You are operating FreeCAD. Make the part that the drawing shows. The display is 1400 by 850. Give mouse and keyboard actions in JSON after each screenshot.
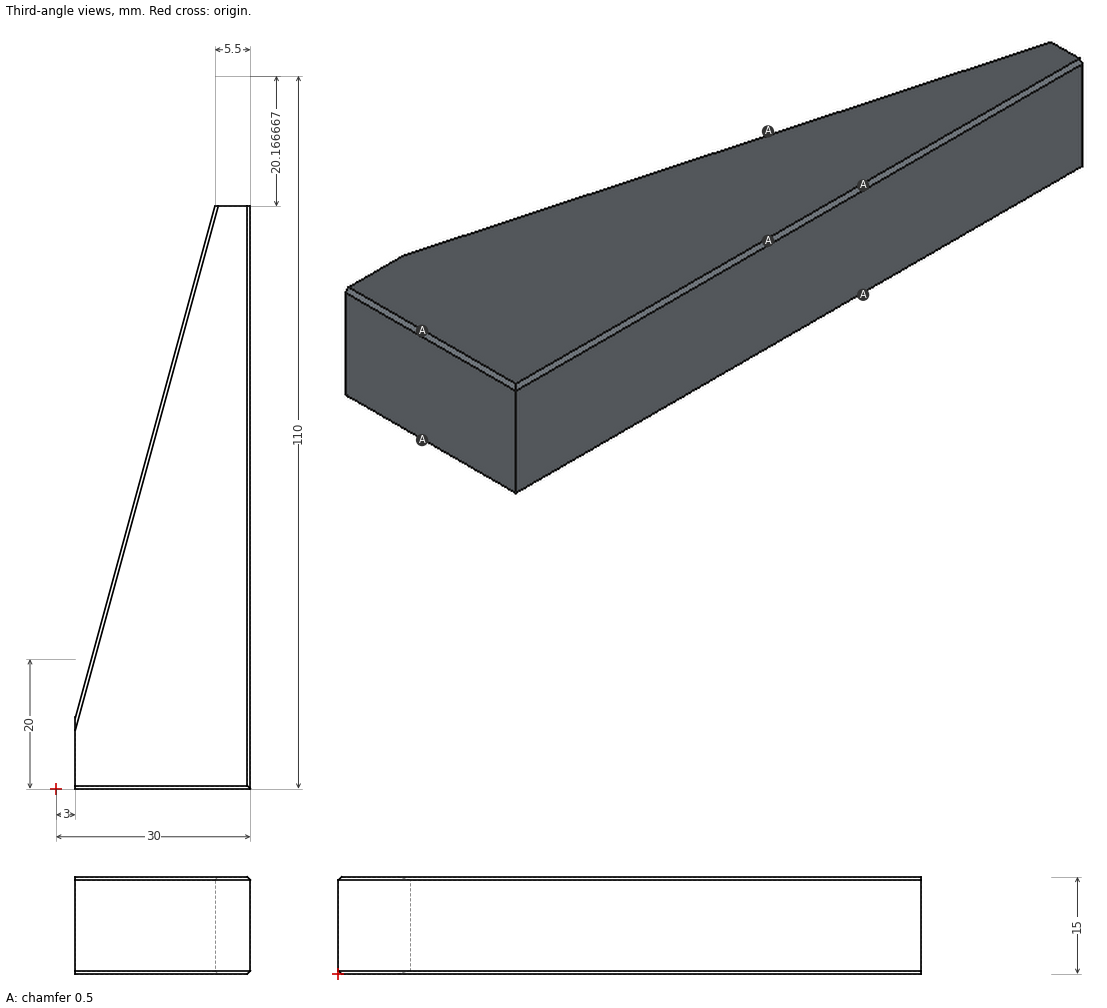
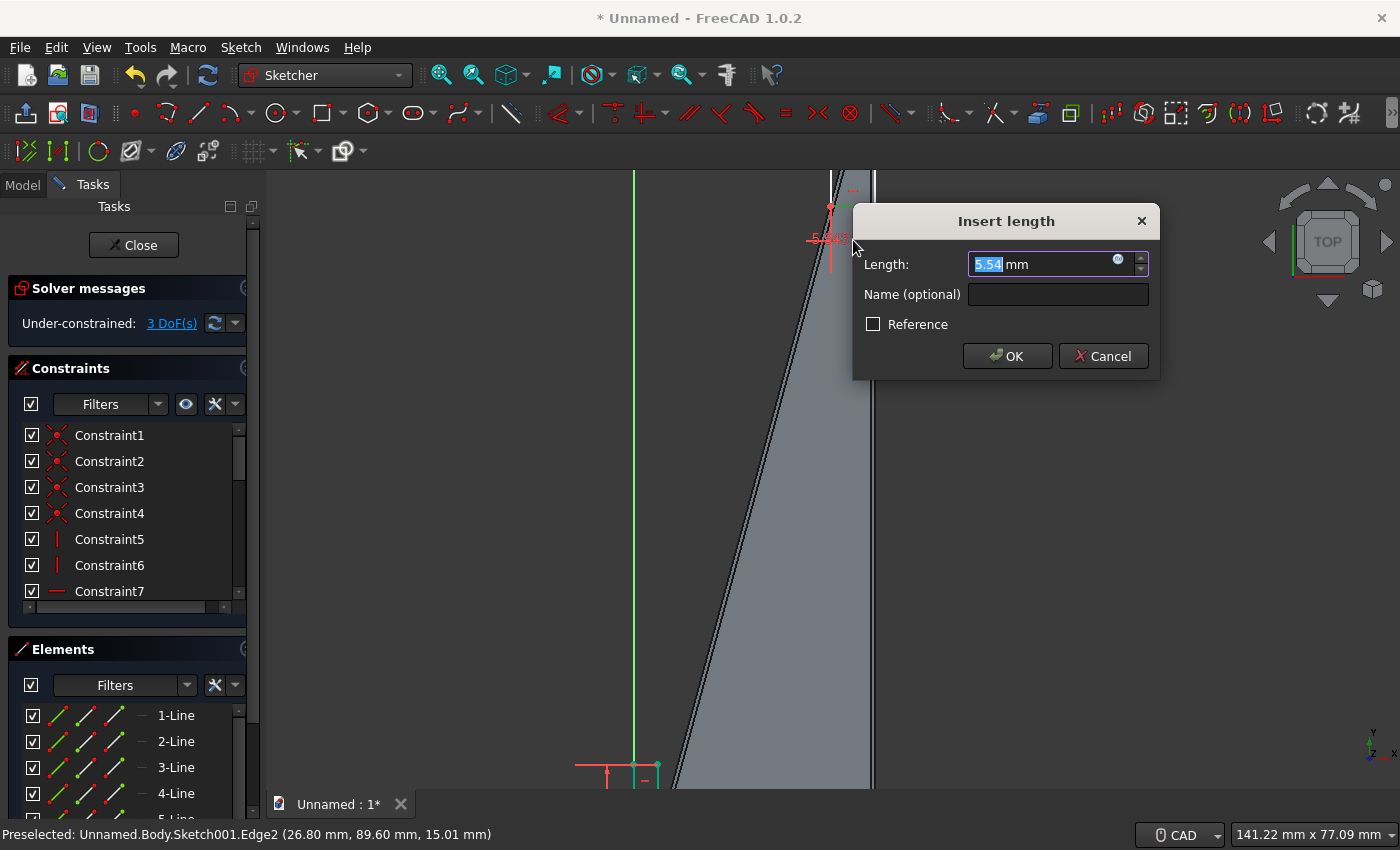
{"action": "type", "text": "5.5"}
{"action": "key", "text": "Return"}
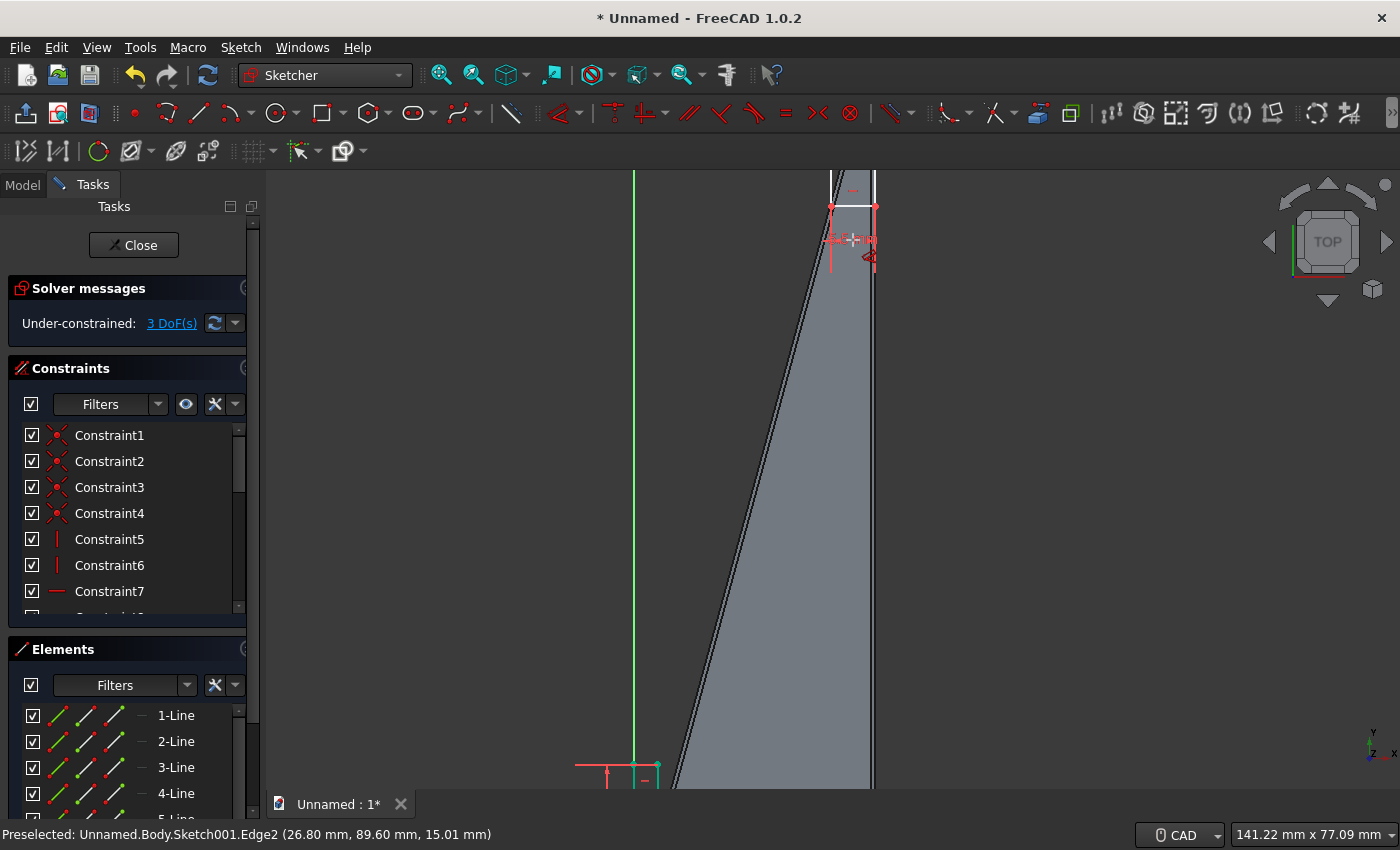
{"action": "left_click", "coordinate": [875, 206]}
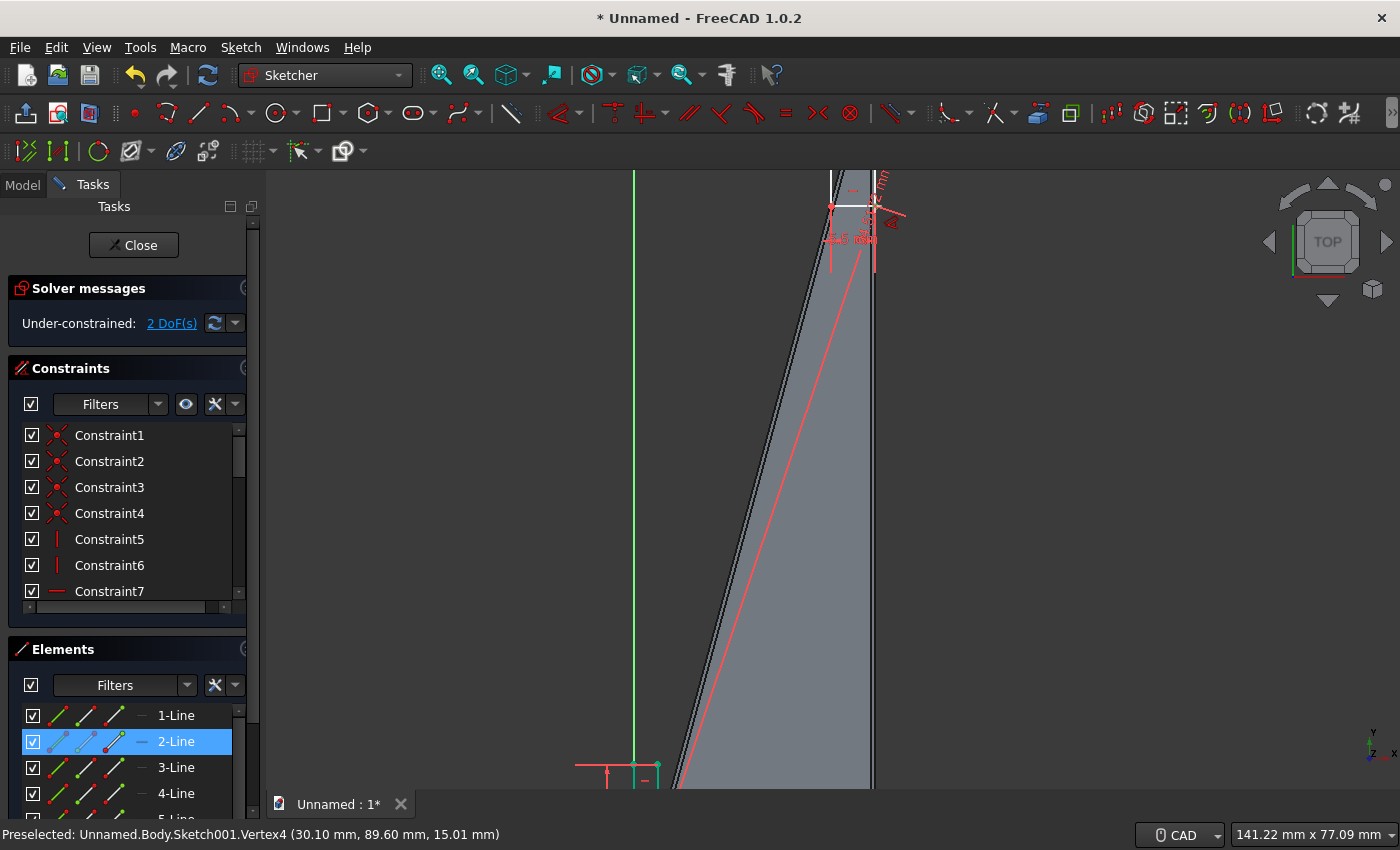
{"action": "key", "text": "Escape"}
{"action": "key", "text": "Escape"}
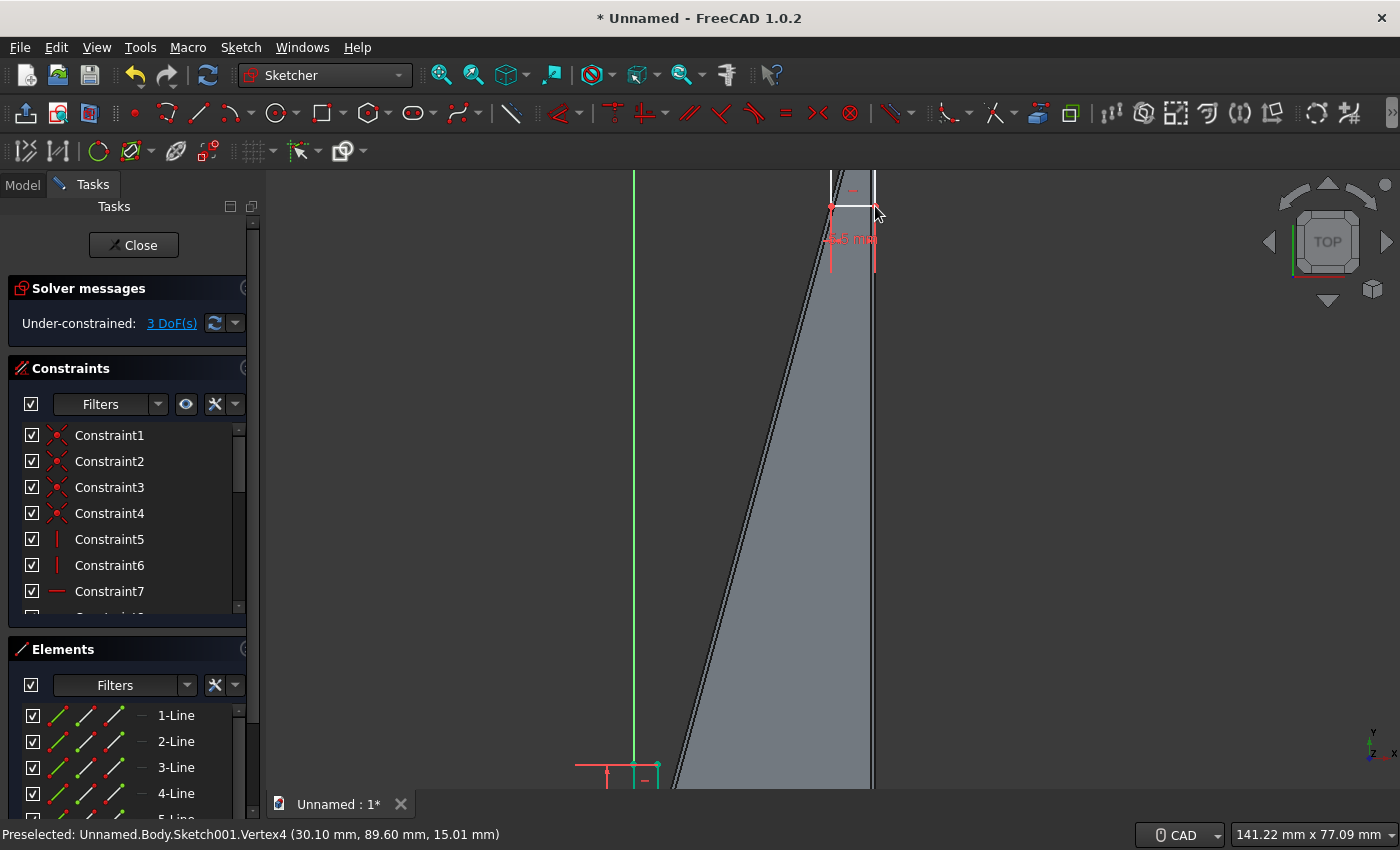
{"action": "left_click", "coordinate": [875, 206]}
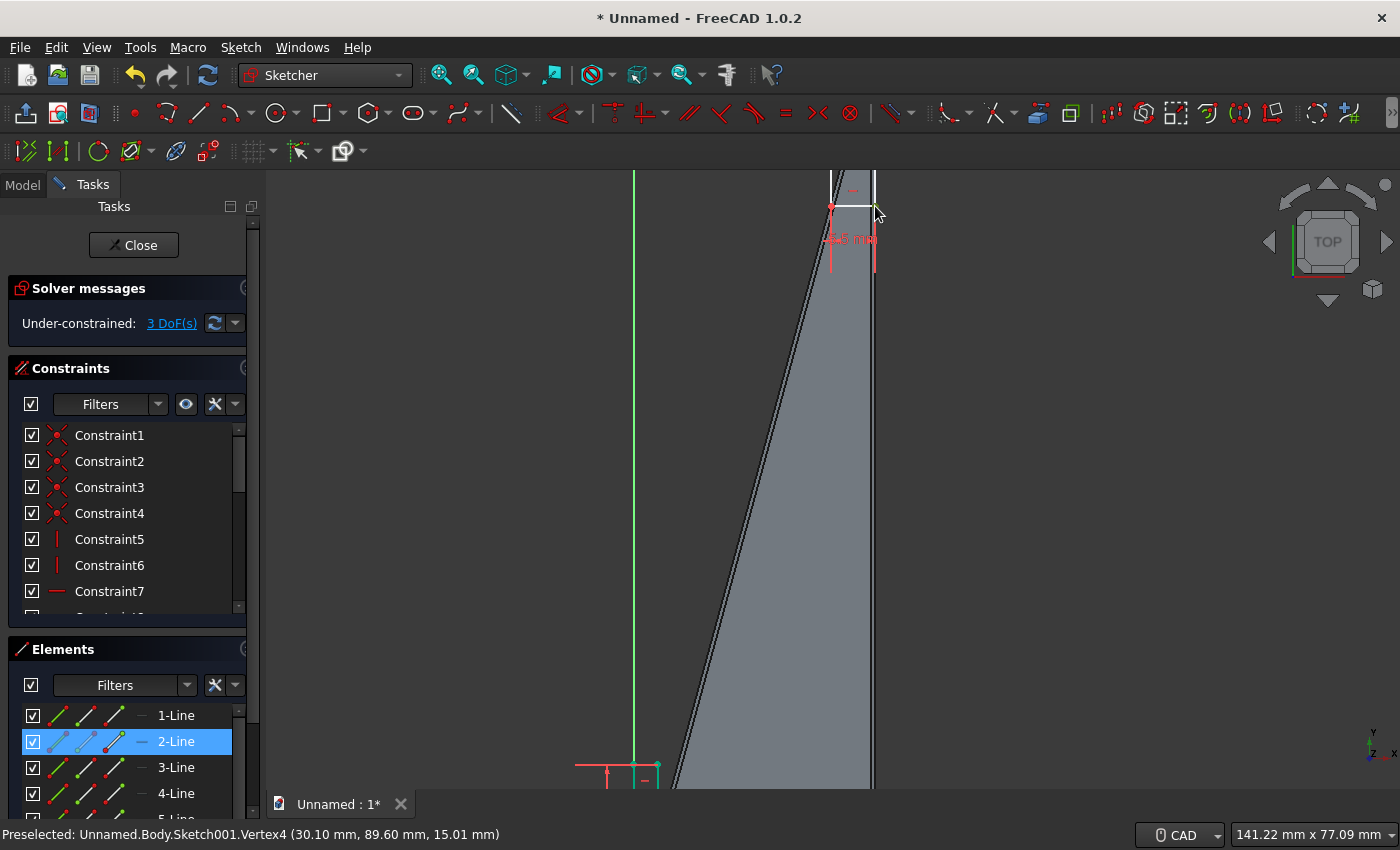
{"action": "key", "text": "l"}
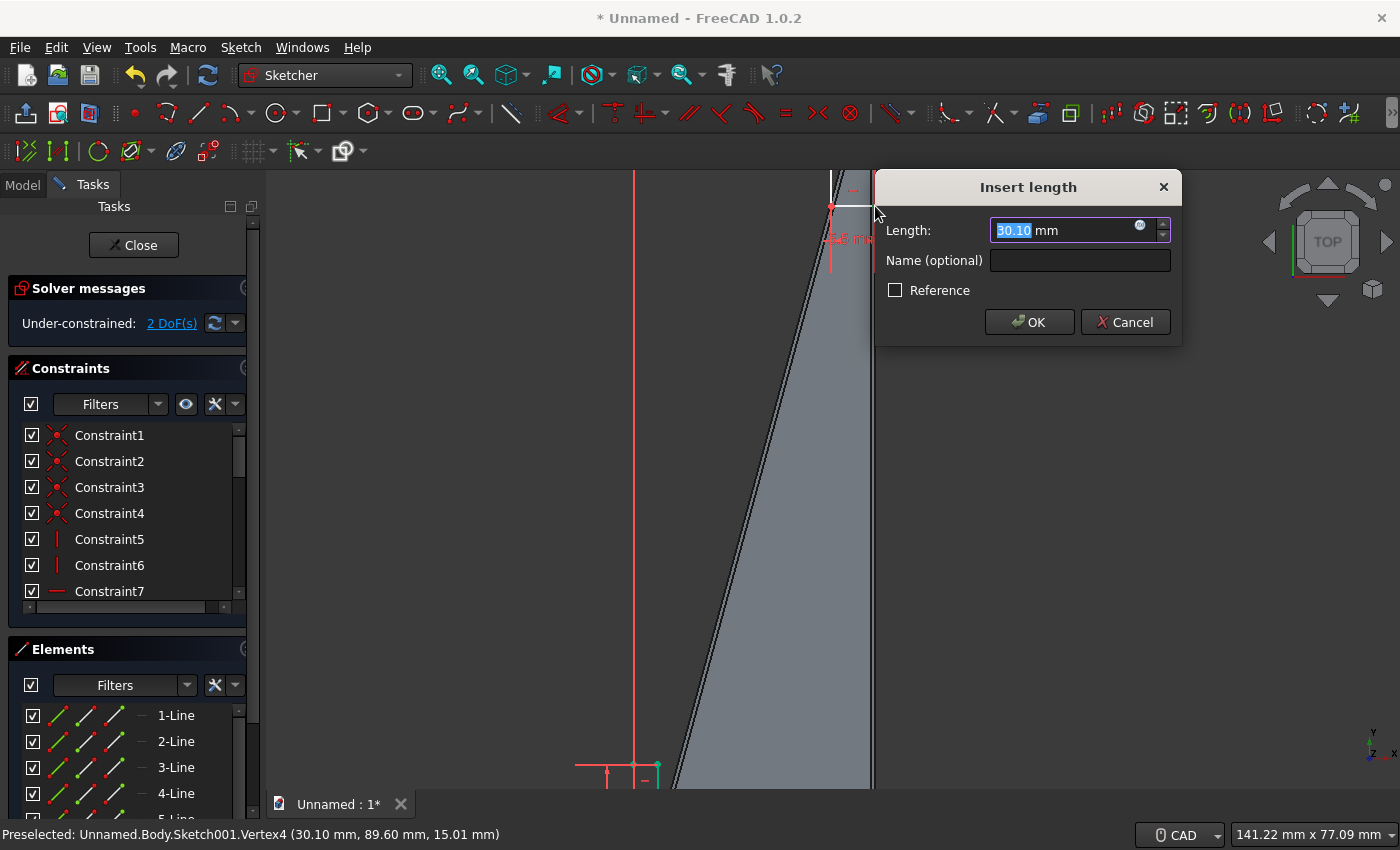
{"action": "type", "text": "30"}
{"action": "key", "text": "Return"}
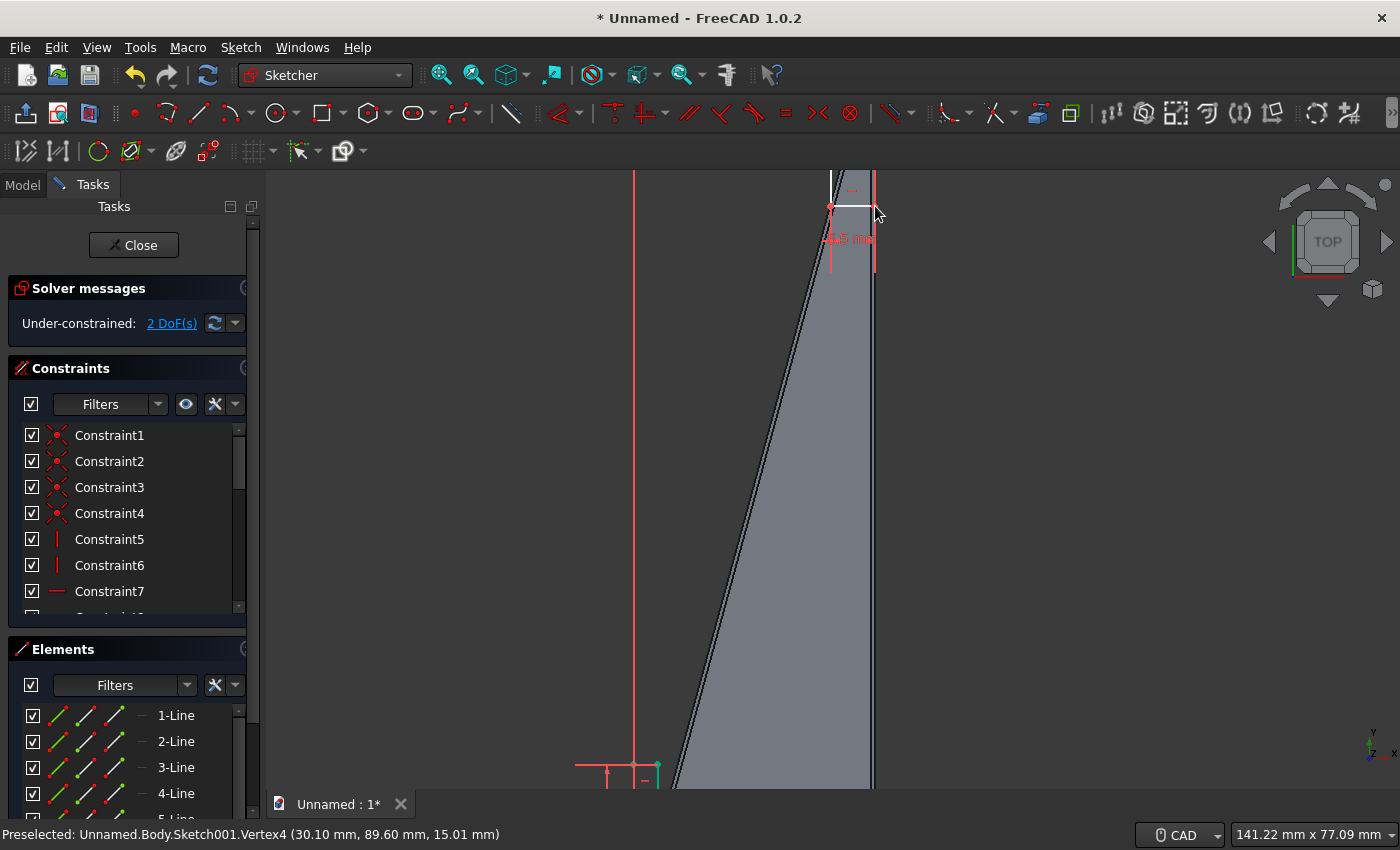
{"action": "scroll", "coordinate": [773, 476], "scroll_direction": "down", "scroll_amount": 4}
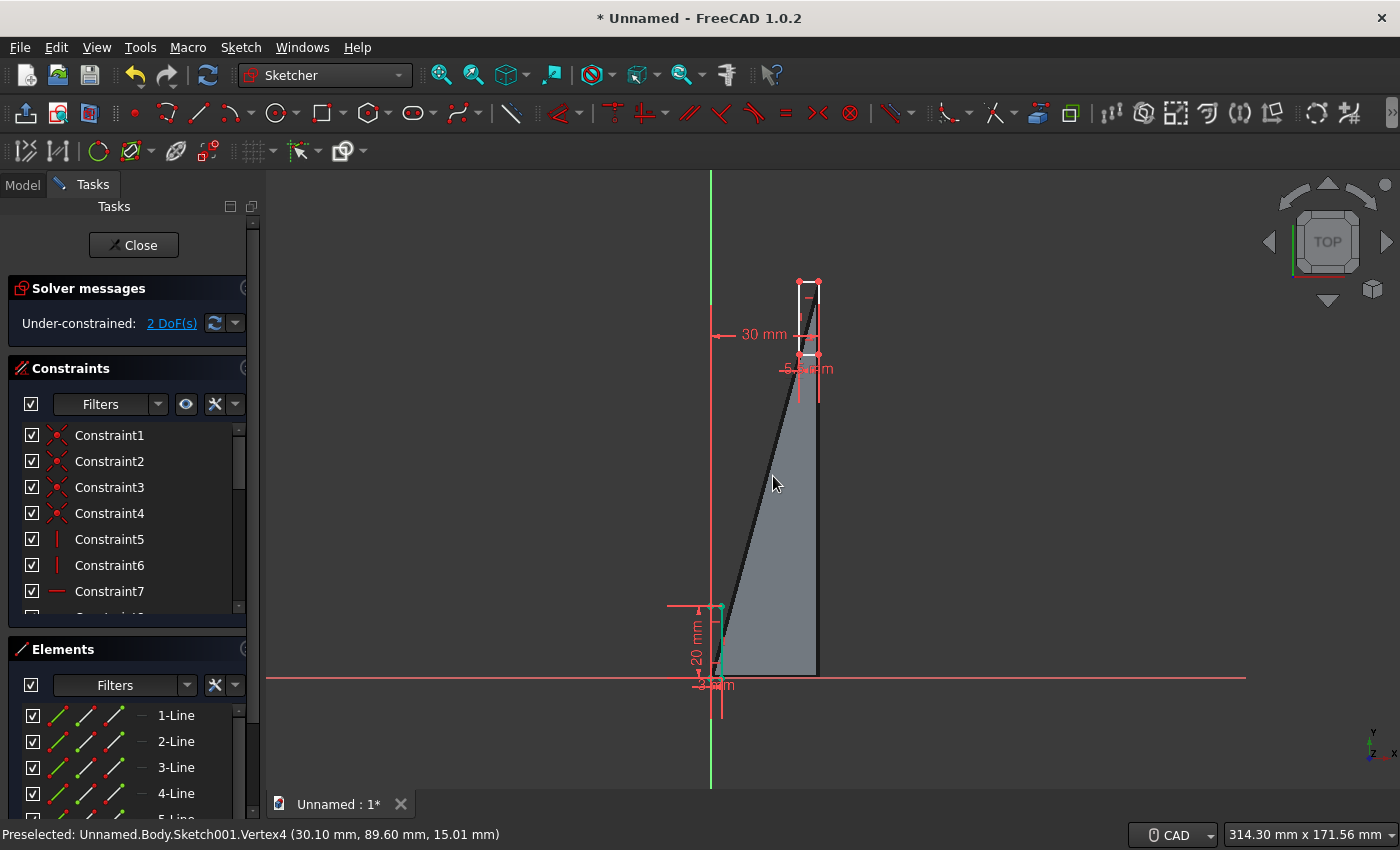
{"action": "left_click", "coordinate": [799, 282]}